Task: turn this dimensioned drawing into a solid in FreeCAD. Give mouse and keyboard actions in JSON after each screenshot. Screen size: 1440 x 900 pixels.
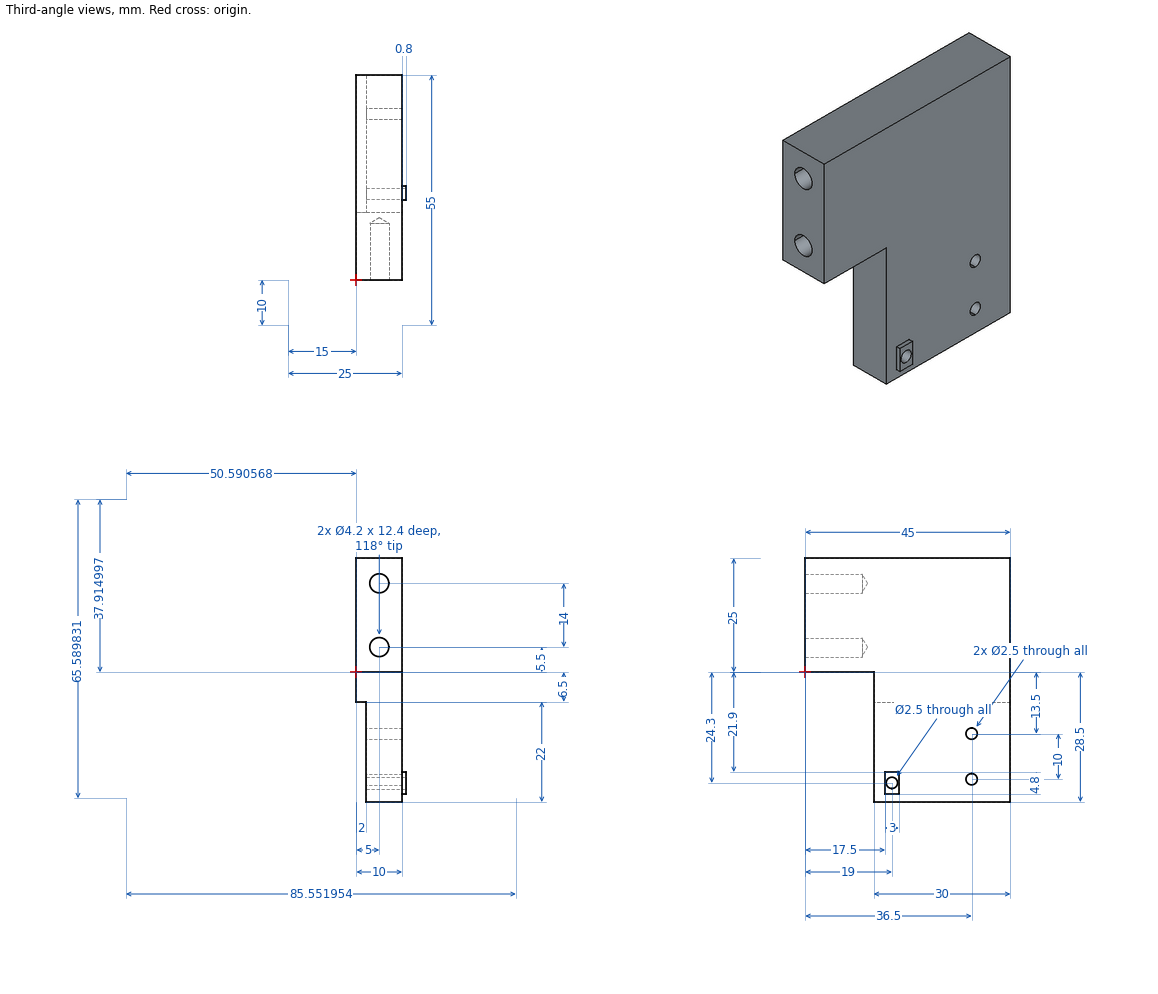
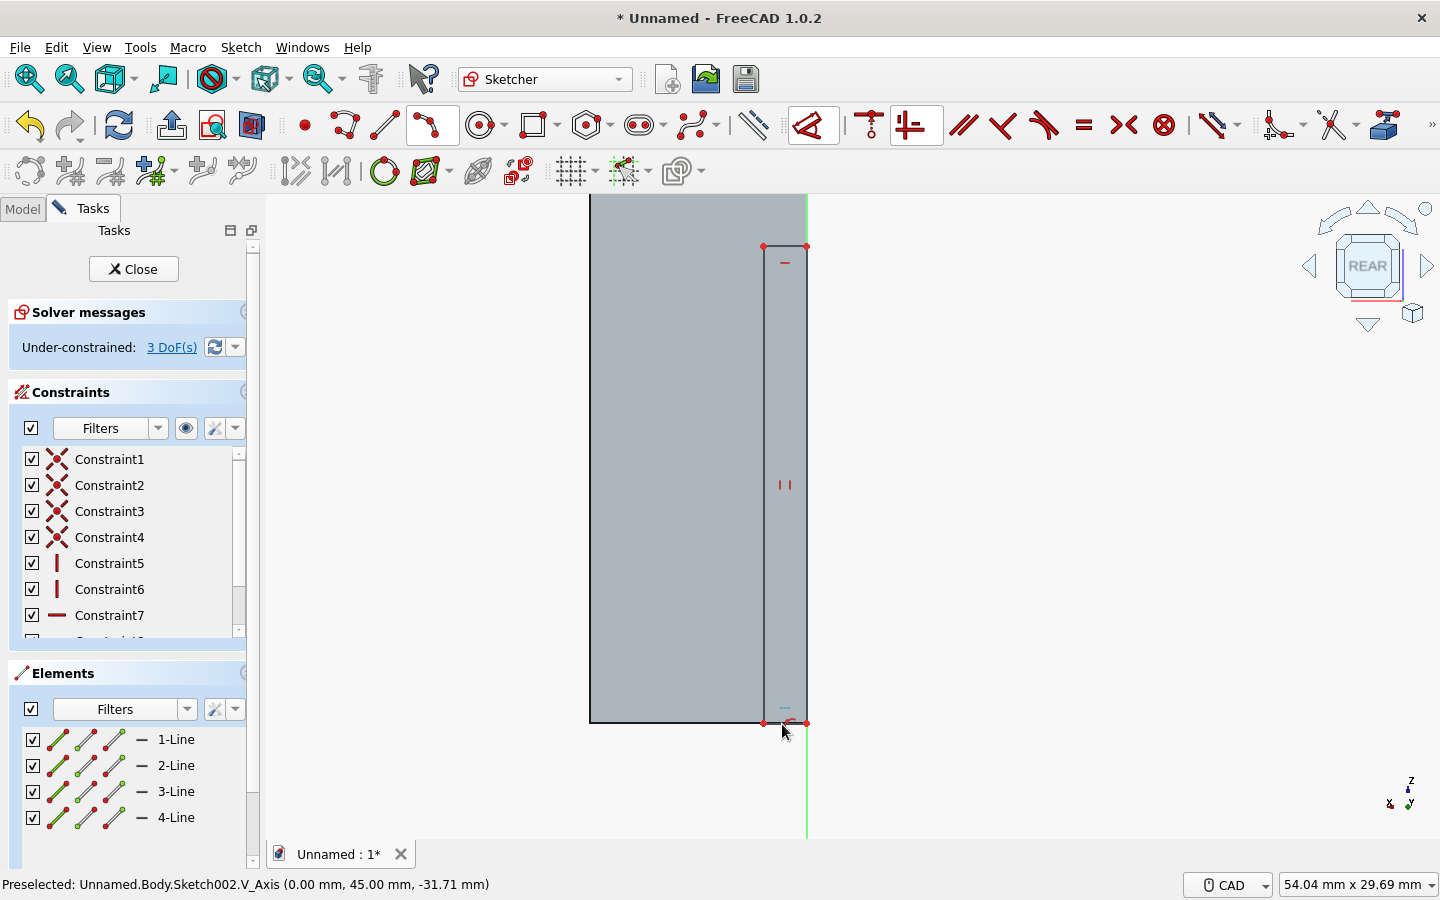
{"action": "left_click", "coordinate": [781, 724]}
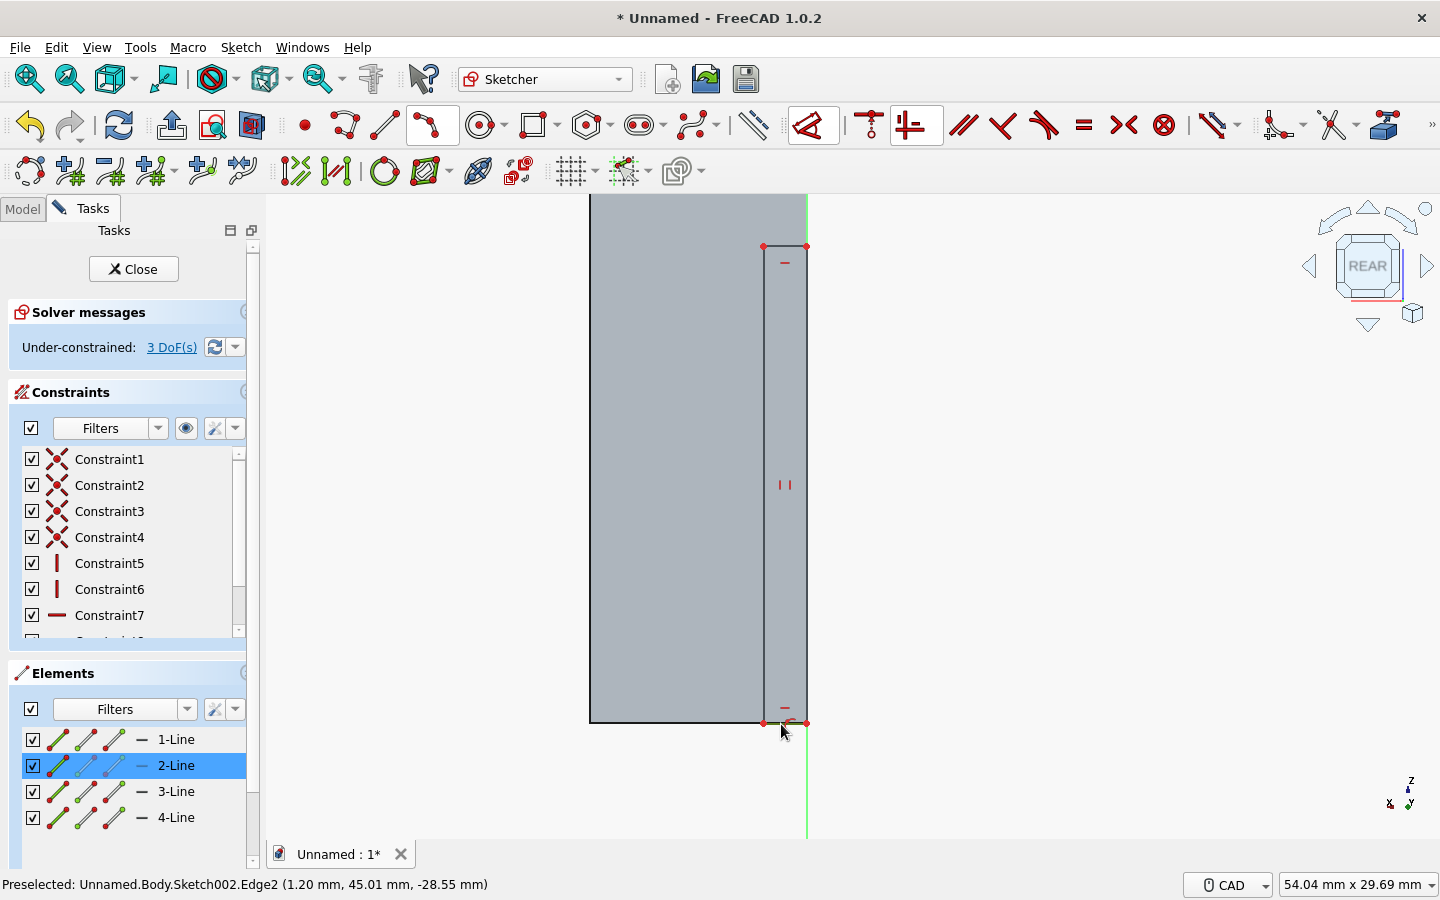
{"action": "left_click", "coordinate": [834, 126]}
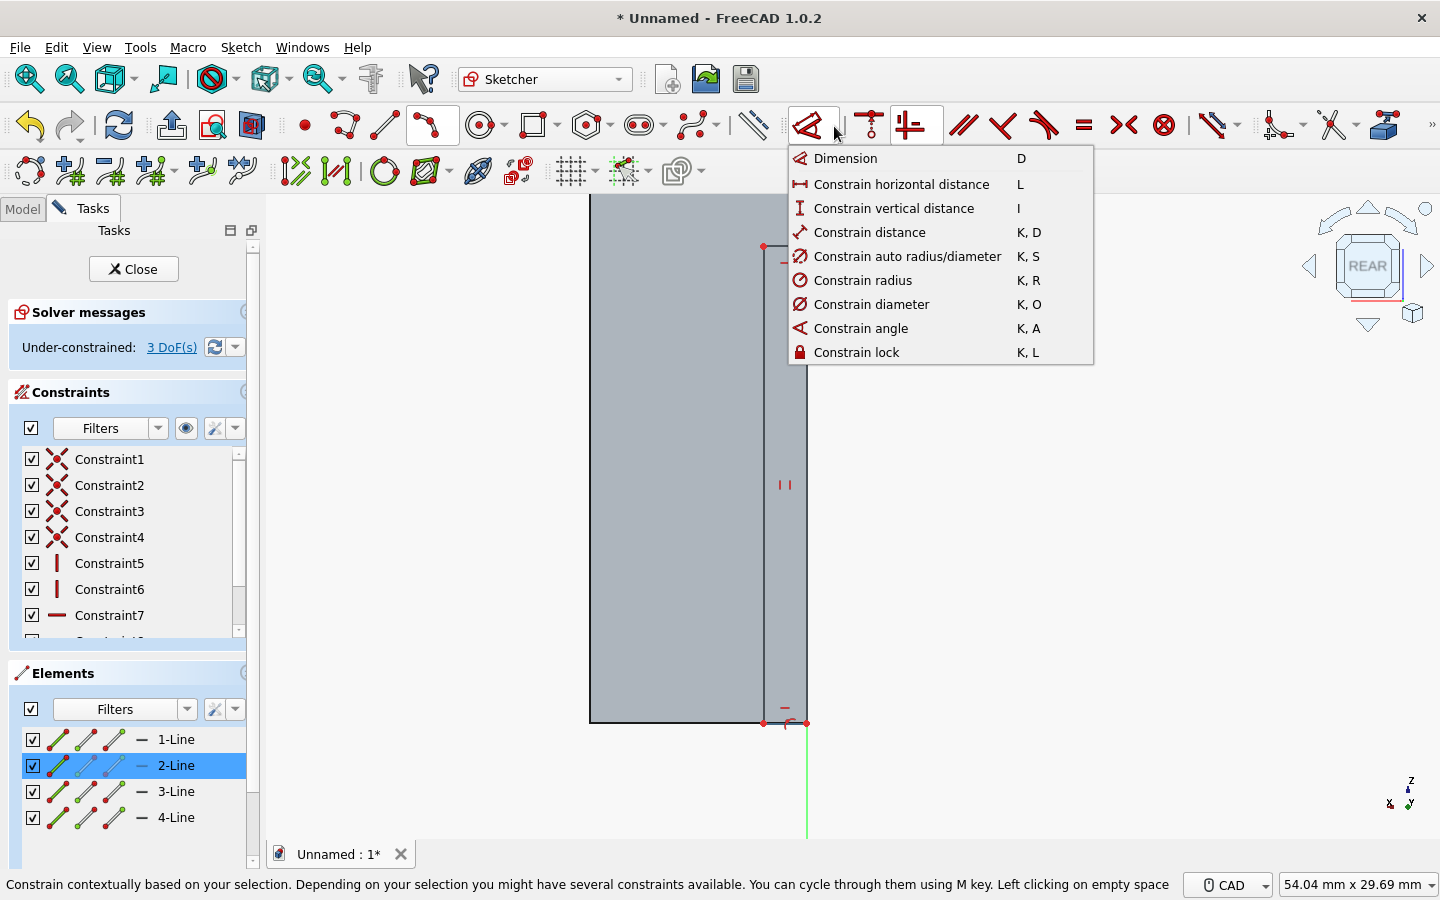
{"action": "left_click", "coordinate": [941, 184]}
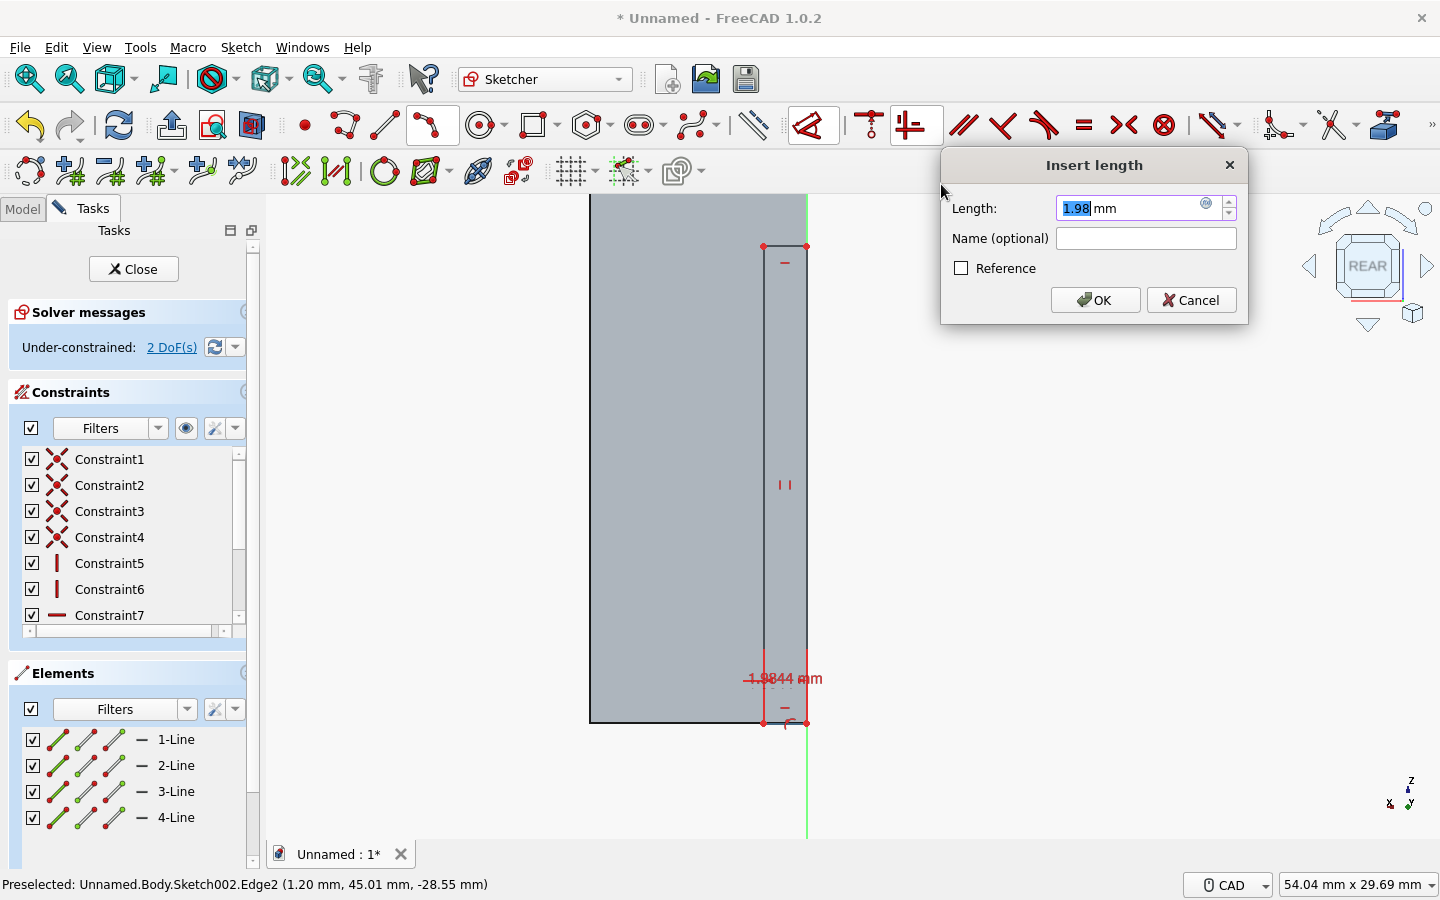
{"action": "type", "text": "2"}
{"action": "key", "text": "Return"}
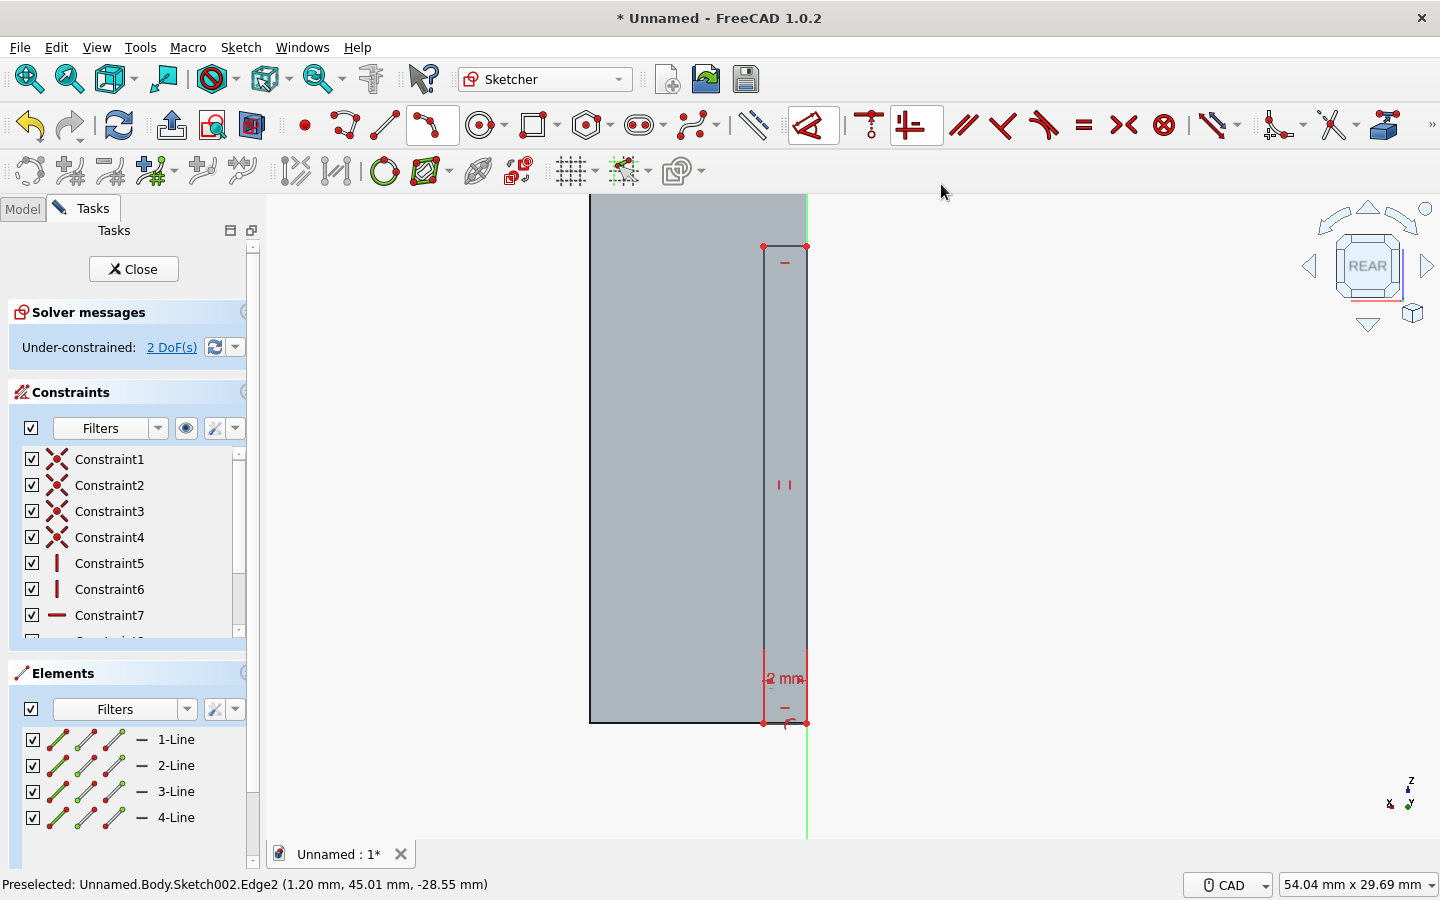
{"action": "left_click", "coordinate": [764, 389]}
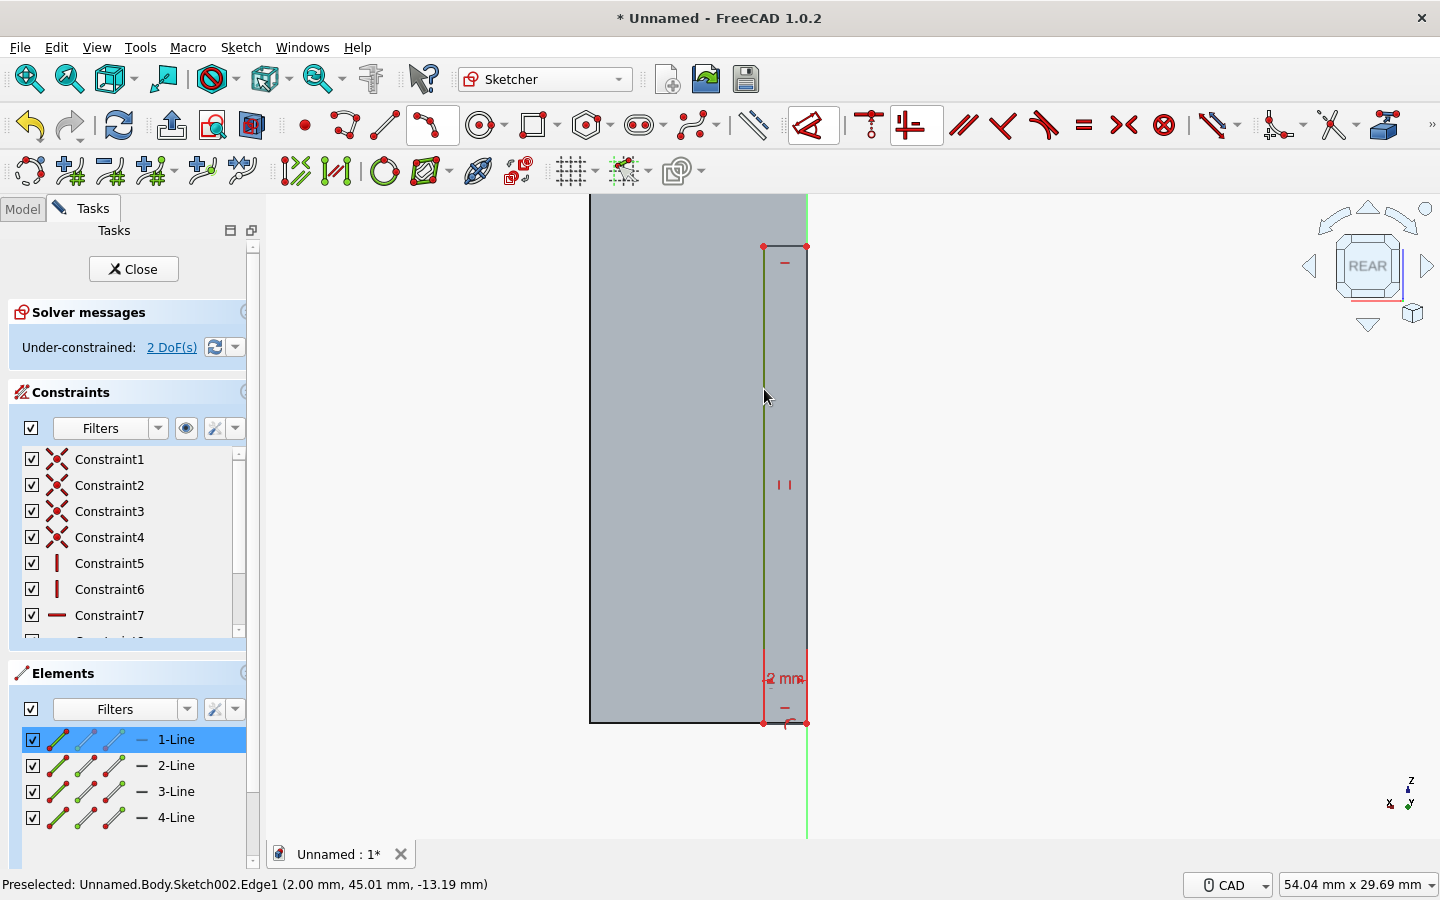
{"action": "left_click", "coordinate": [834, 126]}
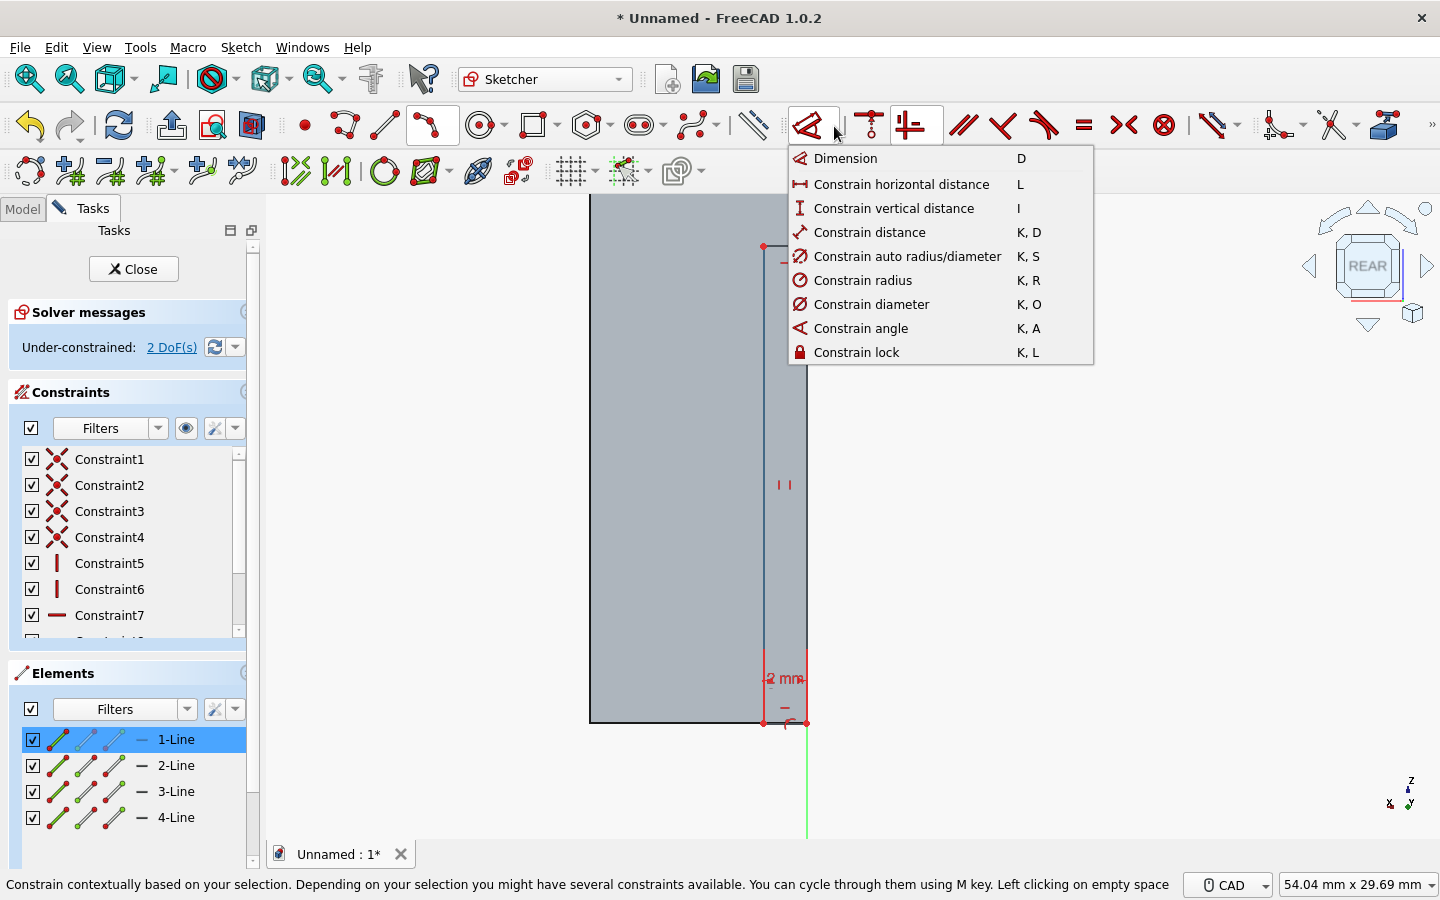
{"action": "left_click", "coordinate": [941, 208]}